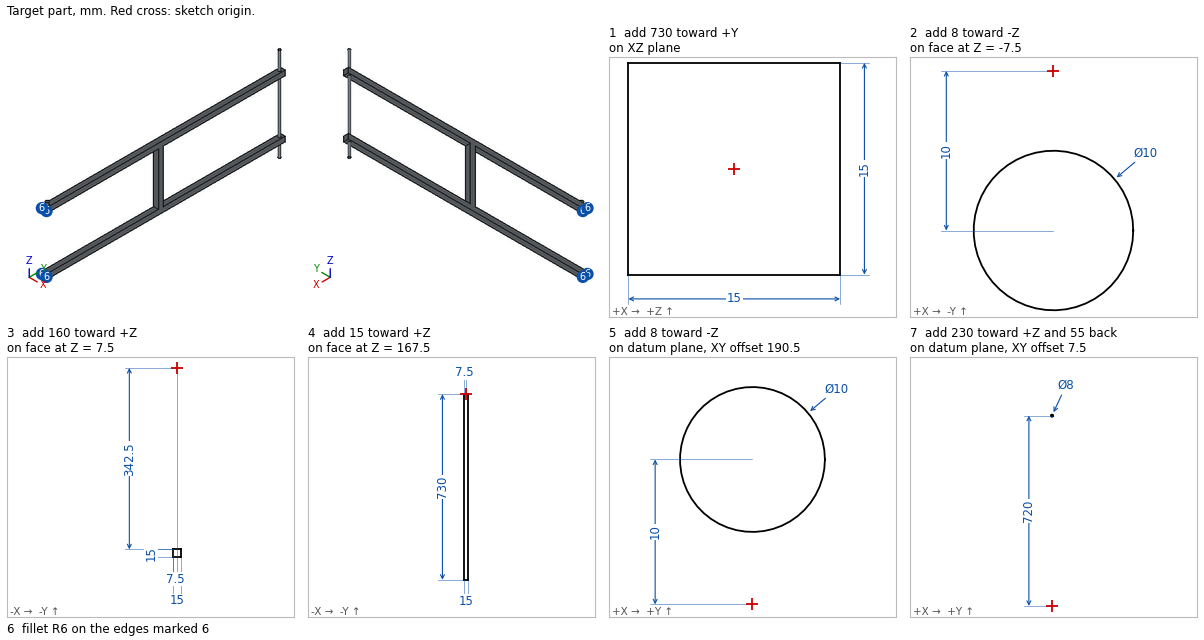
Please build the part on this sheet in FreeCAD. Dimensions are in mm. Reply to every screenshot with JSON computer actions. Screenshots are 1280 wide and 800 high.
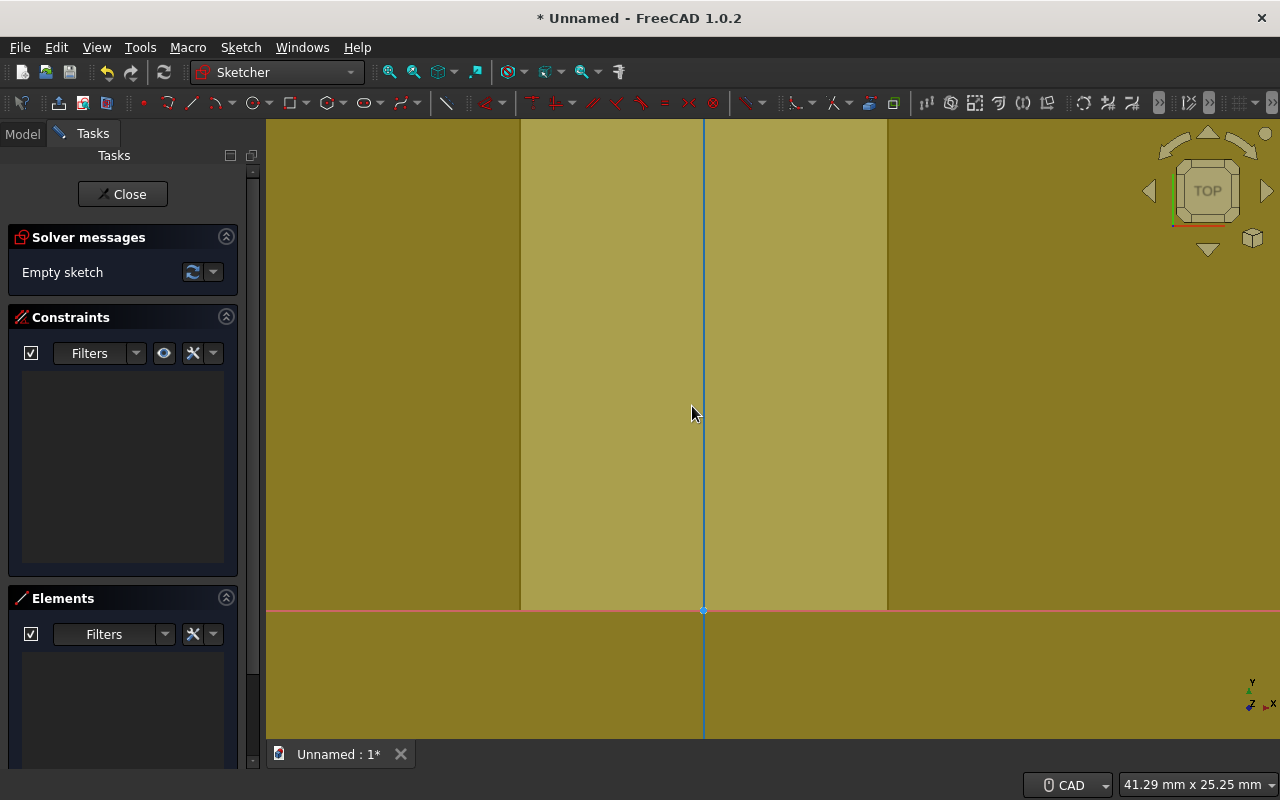
{"action": "left_click", "coordinate": [254, 104]}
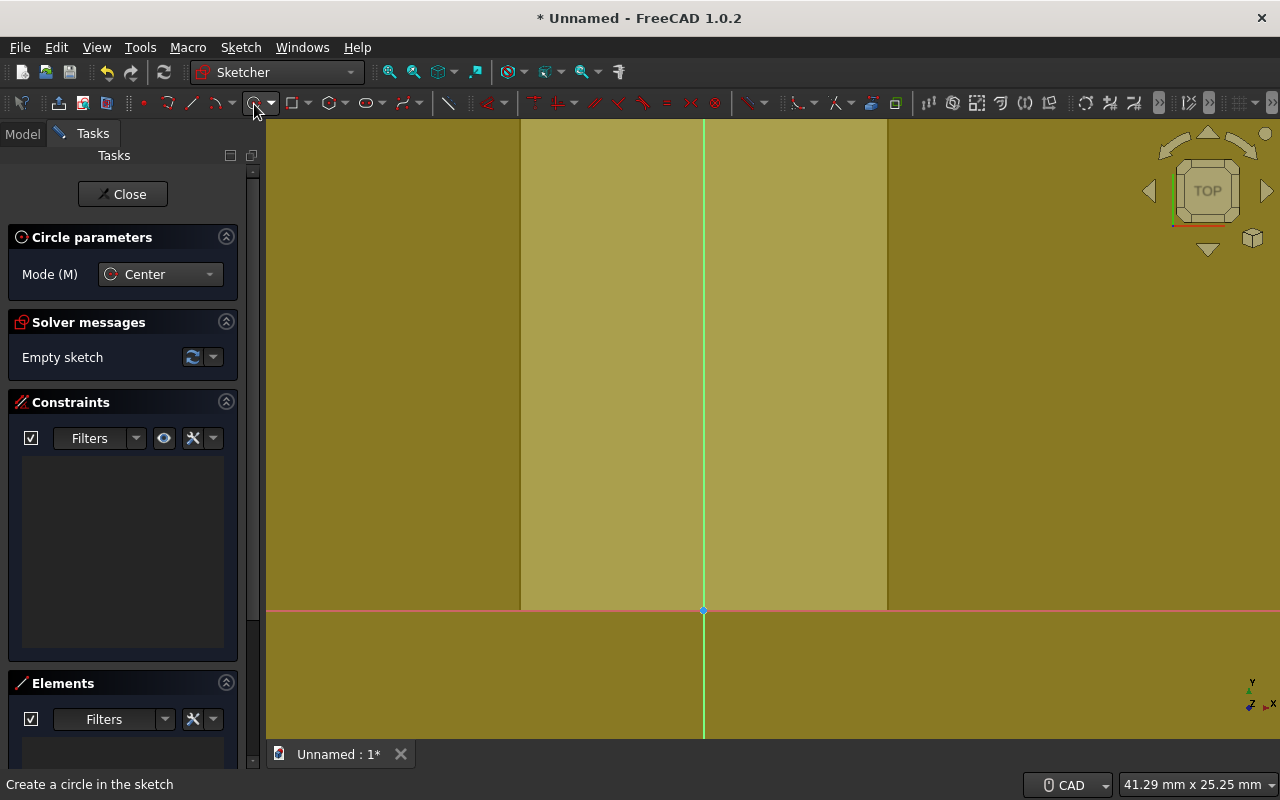
{"action": "left_click", "coordinate": [704, 365]}
{"action": "left_click", "coordinate": [791, 278]}
{"action": "key", "text": "Escape"}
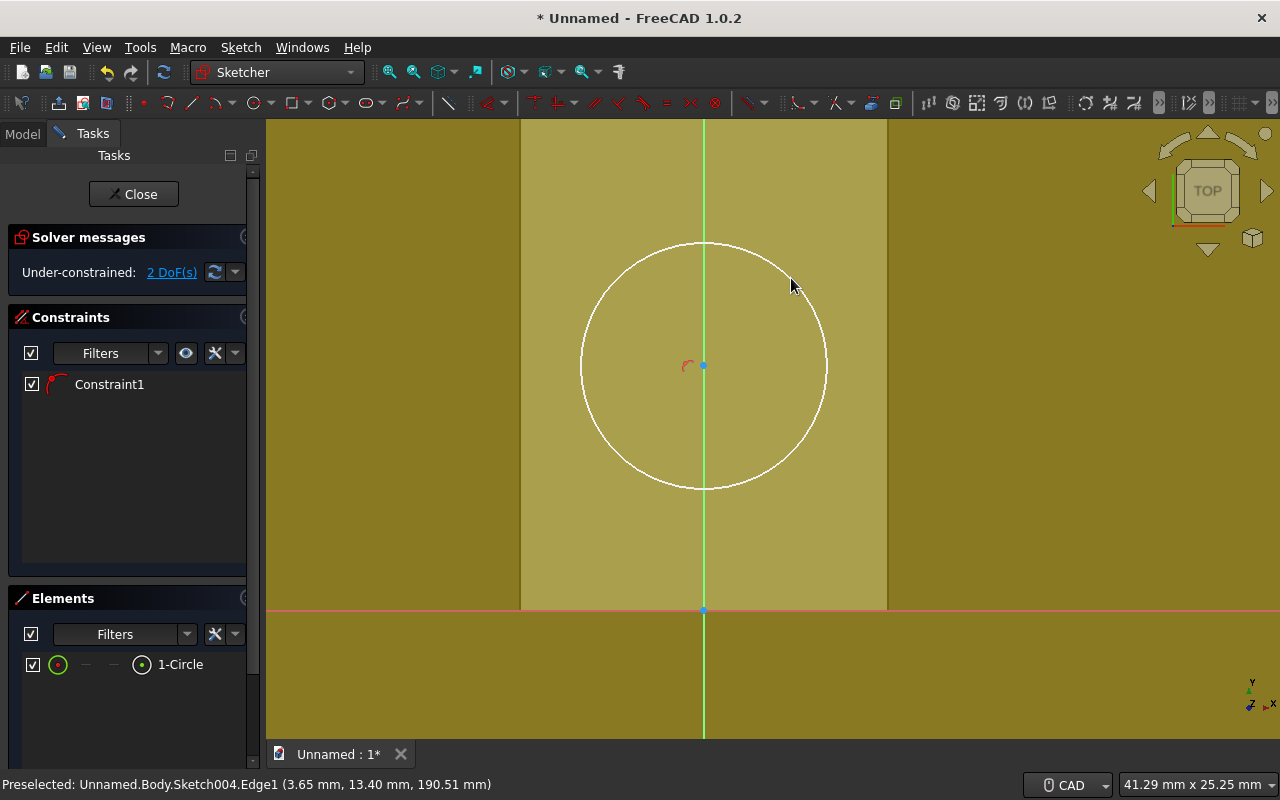
{"action": "left_click", "coordinate": [488, 104]}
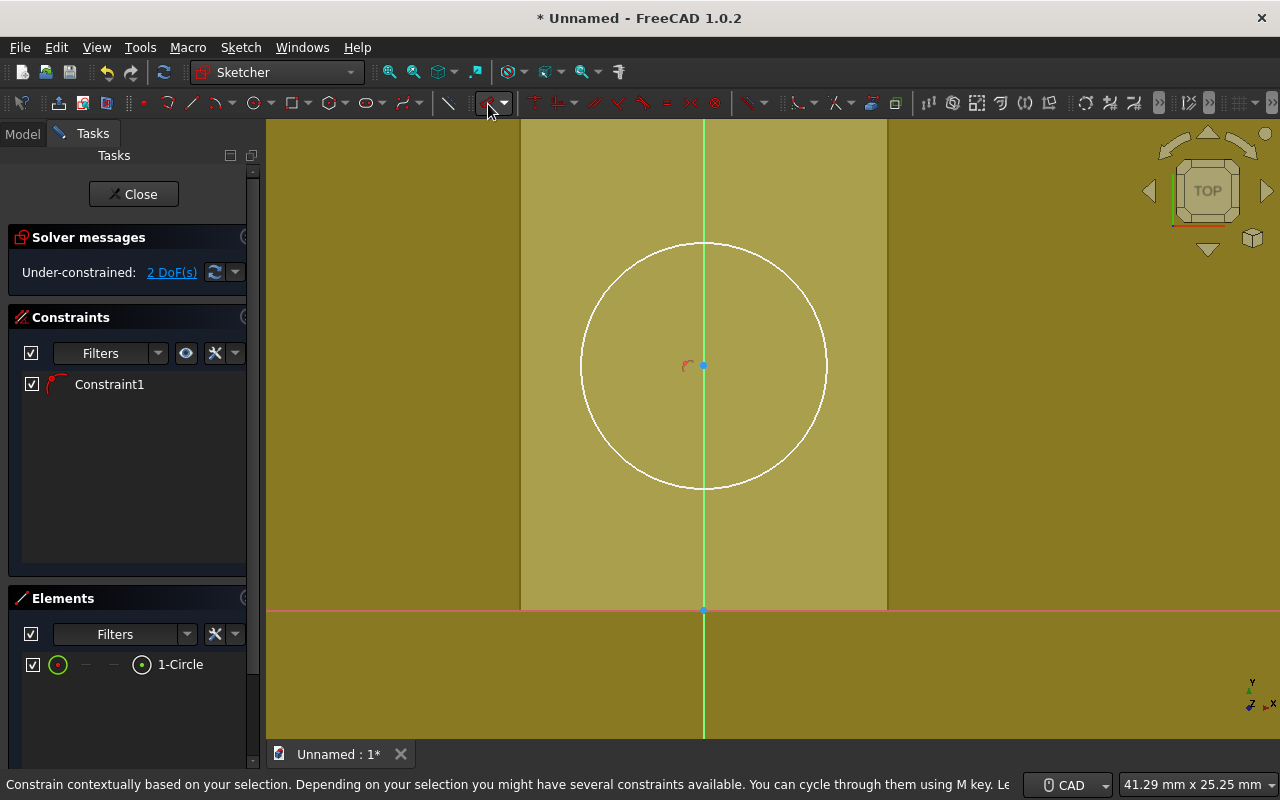
{"action": "left_click", "coordinate": [791, 279]}
{"action": "left_click", "coordinate": [814, 256]}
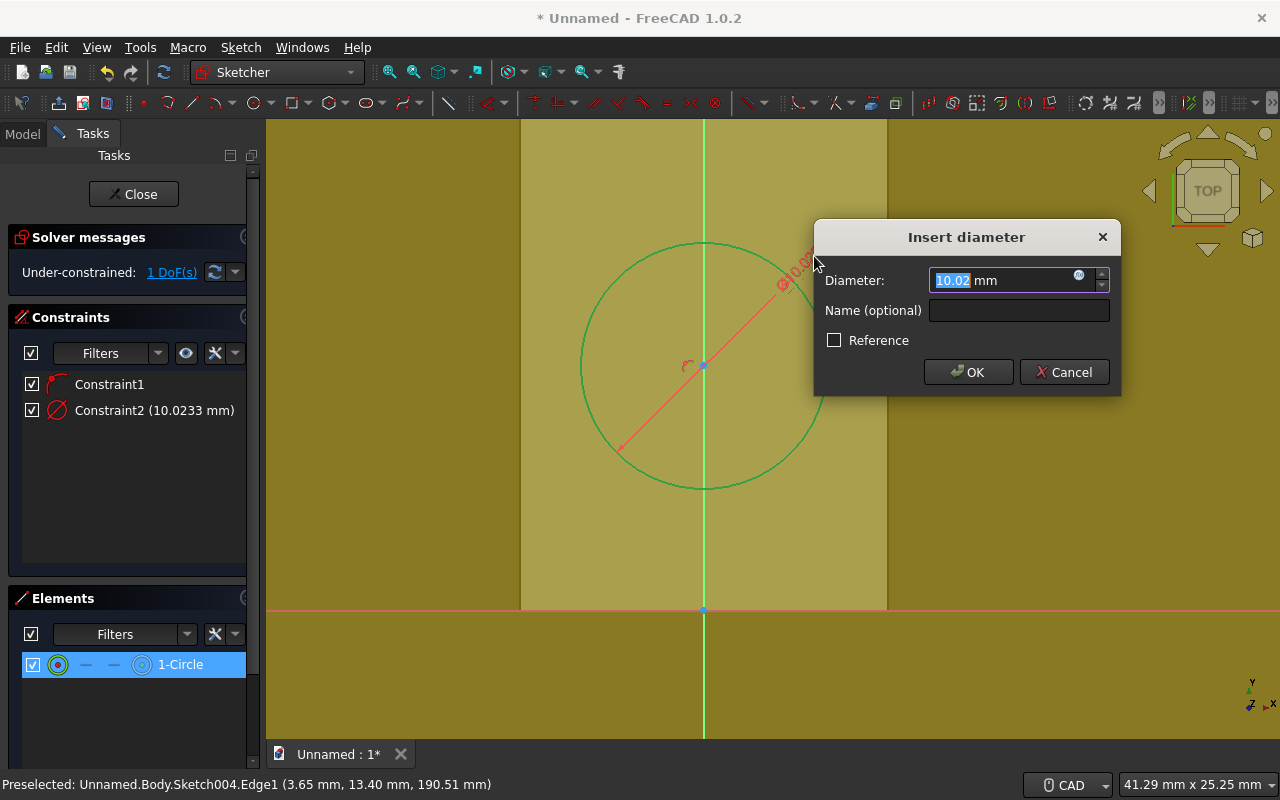
{"action": "type", "text": "10"}
{"action": "key", "text": "Return"}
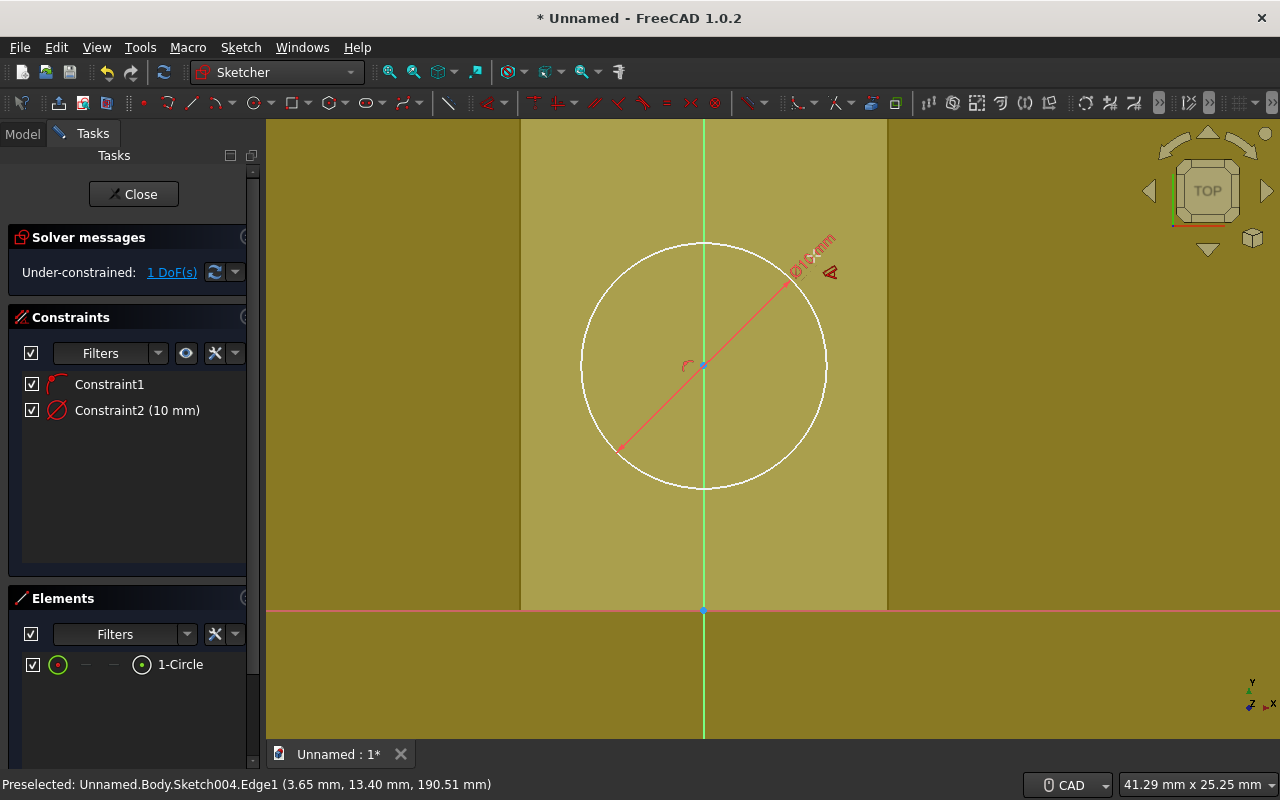
{"action": "left_click", "coordinate": [704, 366]}
{"action": "left_click", "coordinate": [738, 432]}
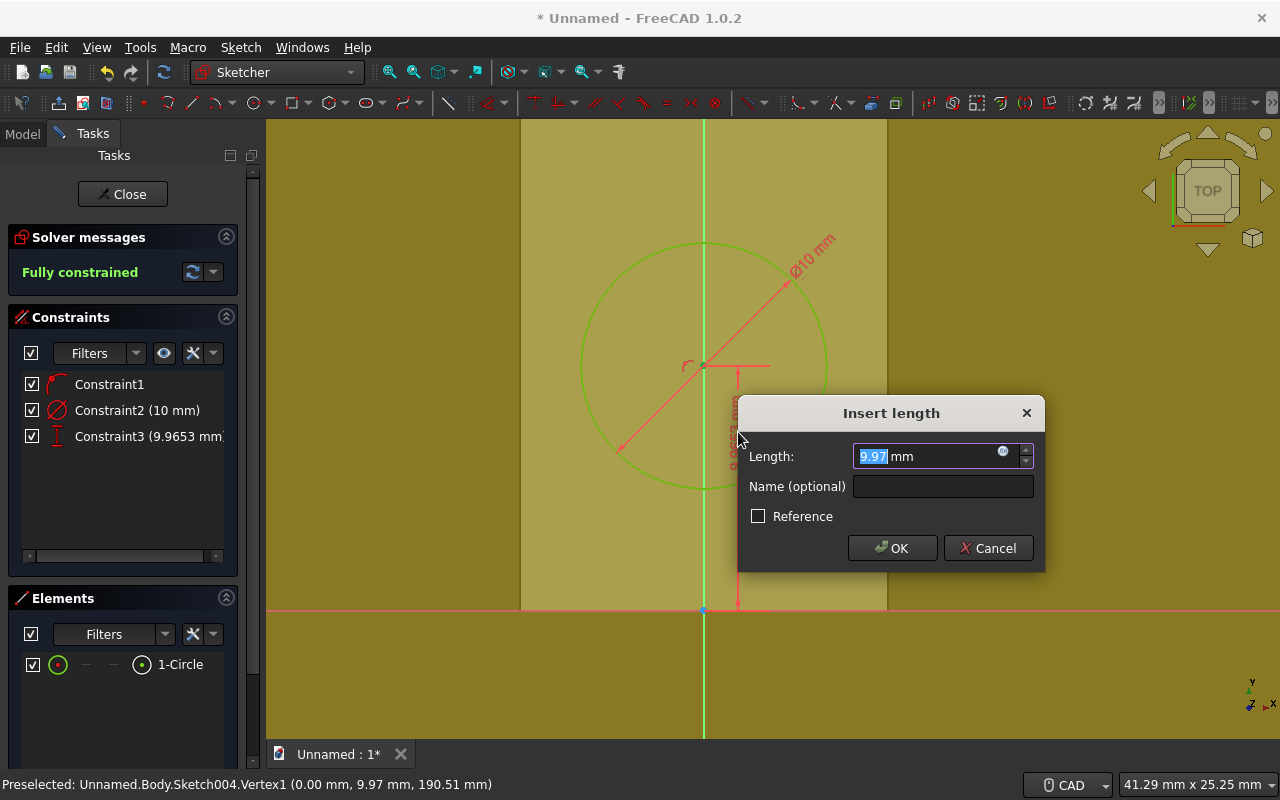
{"action": "type", "text": "10"}
{"action": "key", "text": "Return"}
{"action": "key", "text": "Escape"}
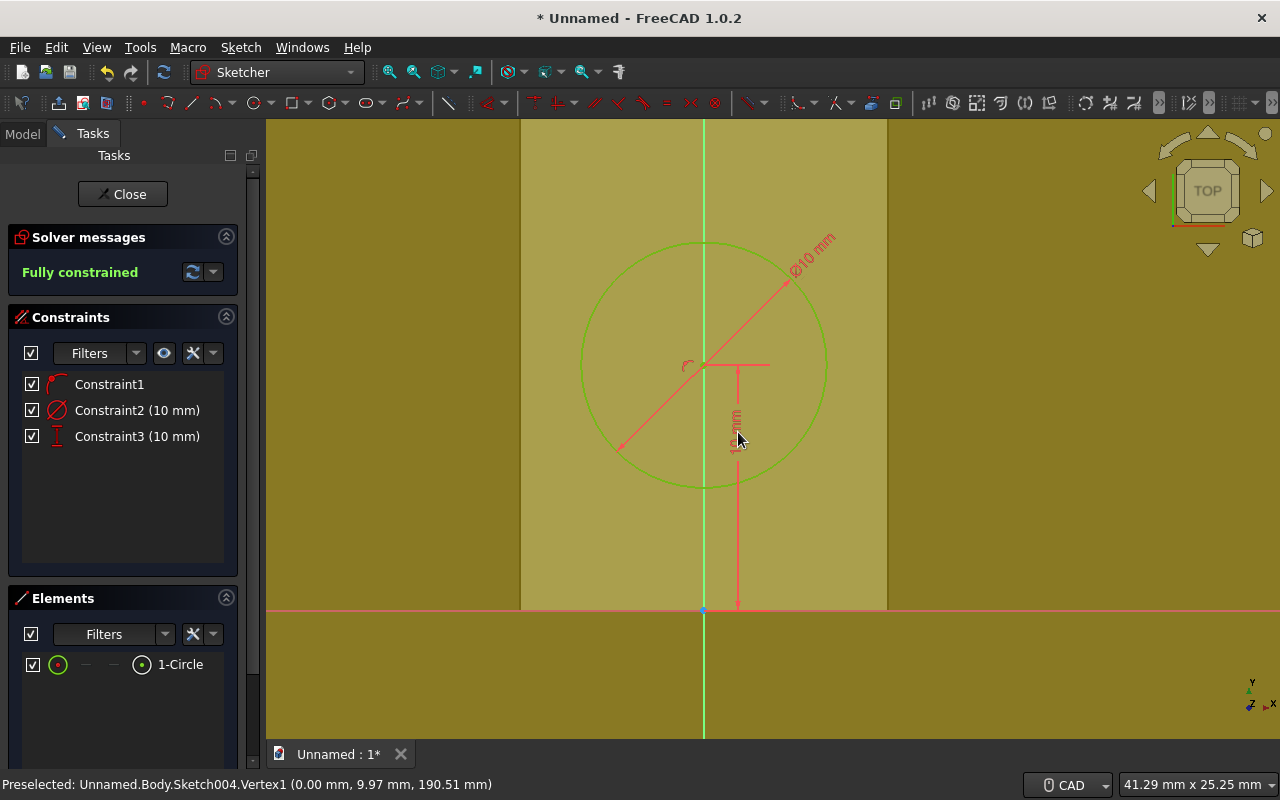
{"action": "left_click", "coordinate": [123, 194]}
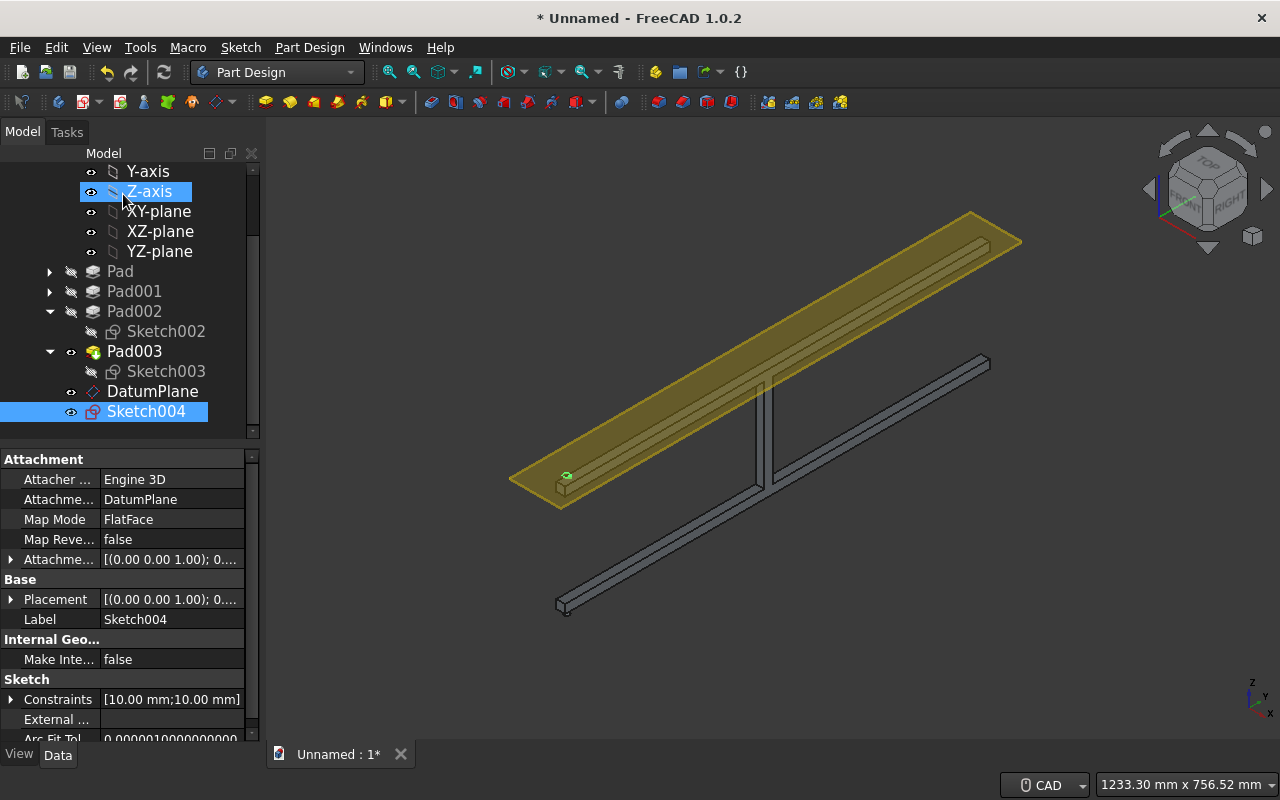
{"action": "left_click", "coordinate": [266, 102]}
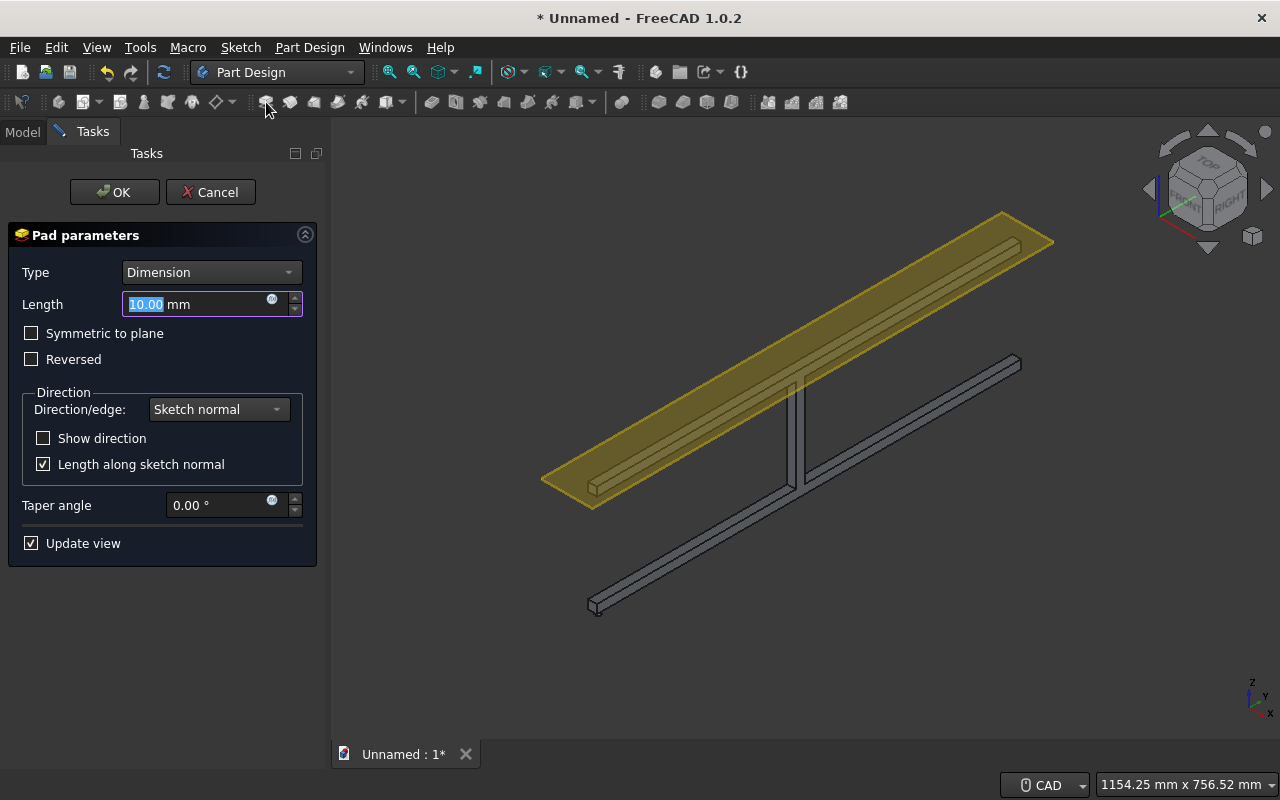
{"action": "type", "text": "8"}
{"action": "key", "text": "Tab"}